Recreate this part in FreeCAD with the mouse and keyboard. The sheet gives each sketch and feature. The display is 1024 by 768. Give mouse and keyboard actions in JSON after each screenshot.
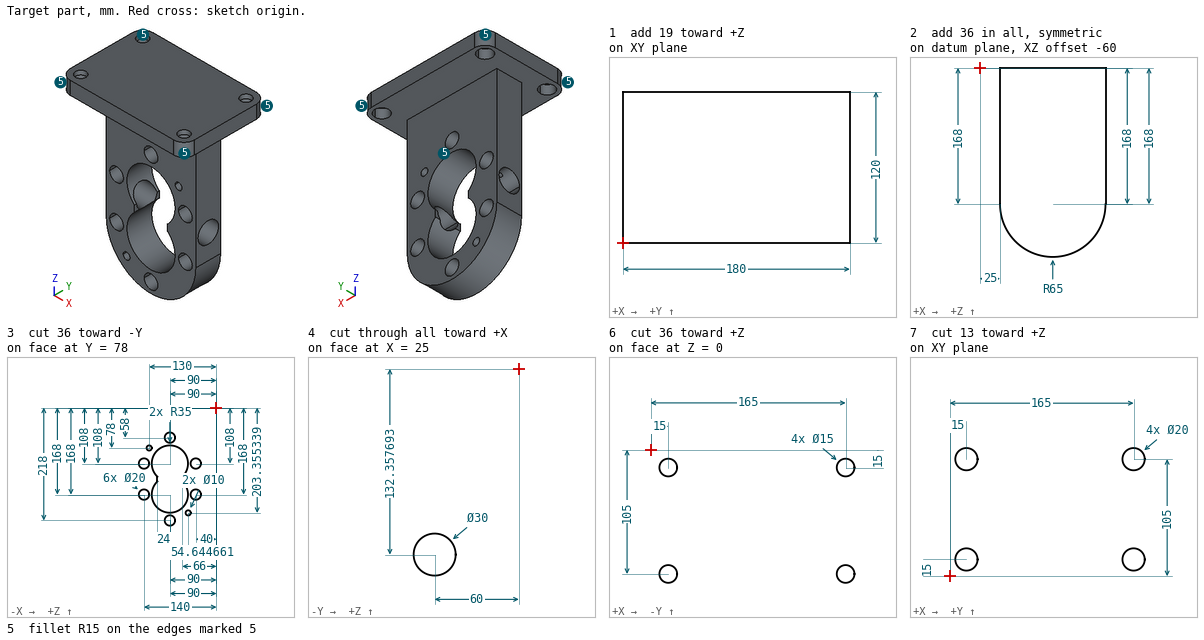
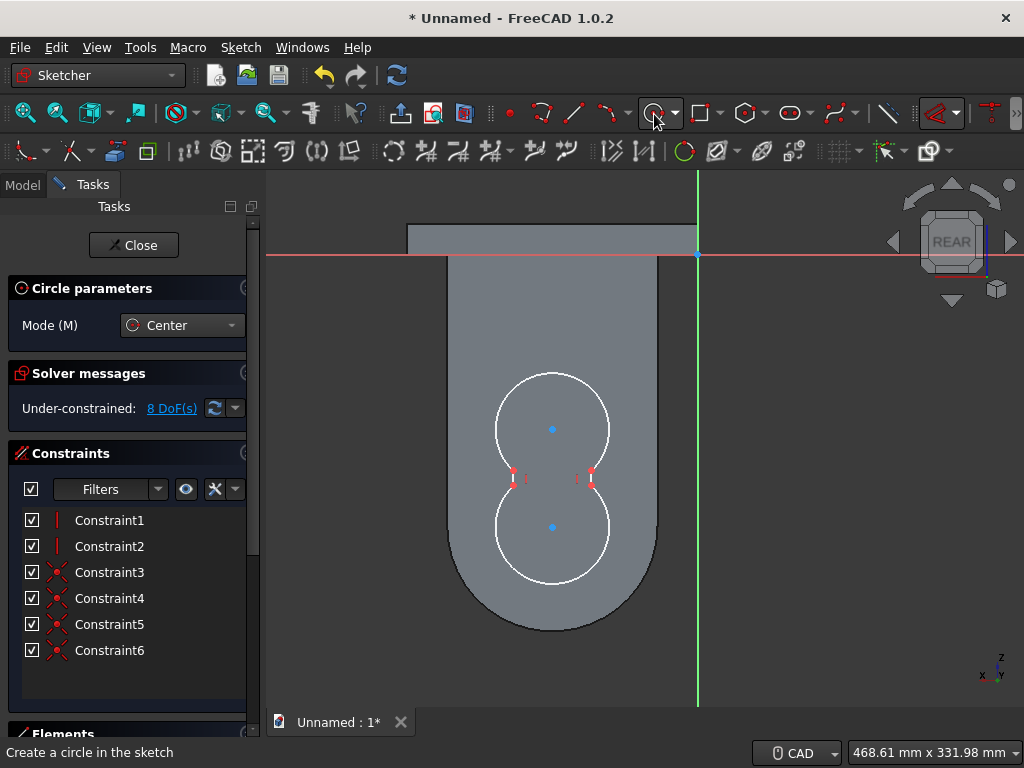
{"action": "scroll", "coordinate": [552, 607], "scroll_direction": "up", "scroll_amount": 2}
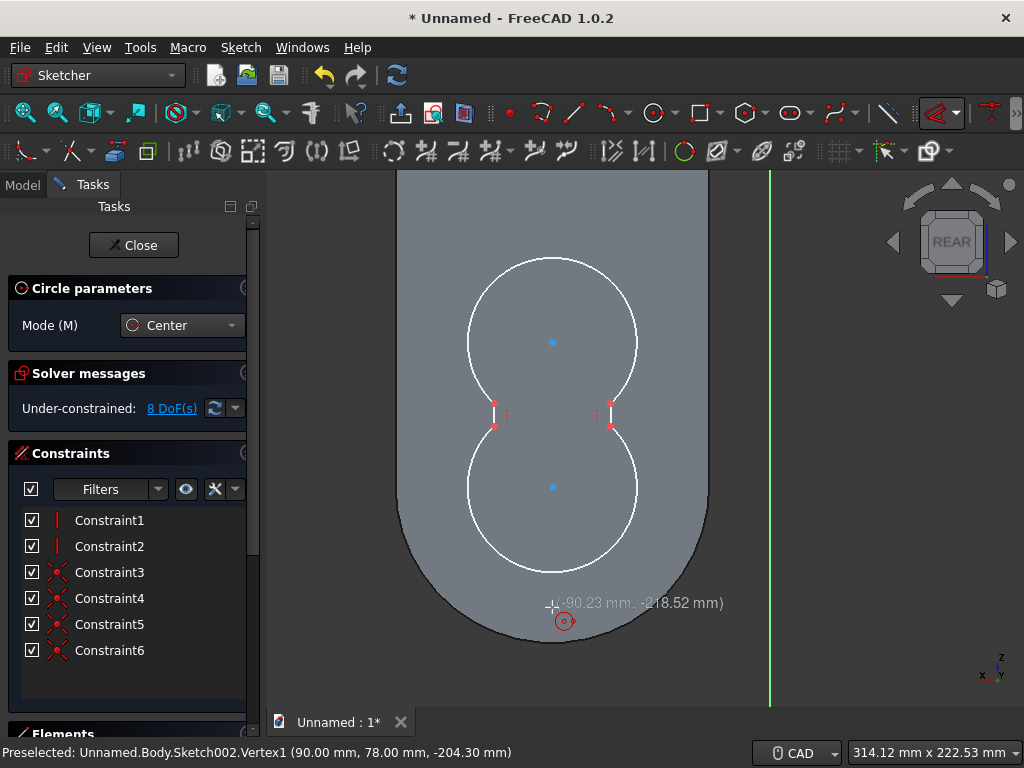
{"action": "left_click", "coordinate": [552, 607]}
{"action": "left_click", "coordinate": [569, 590]}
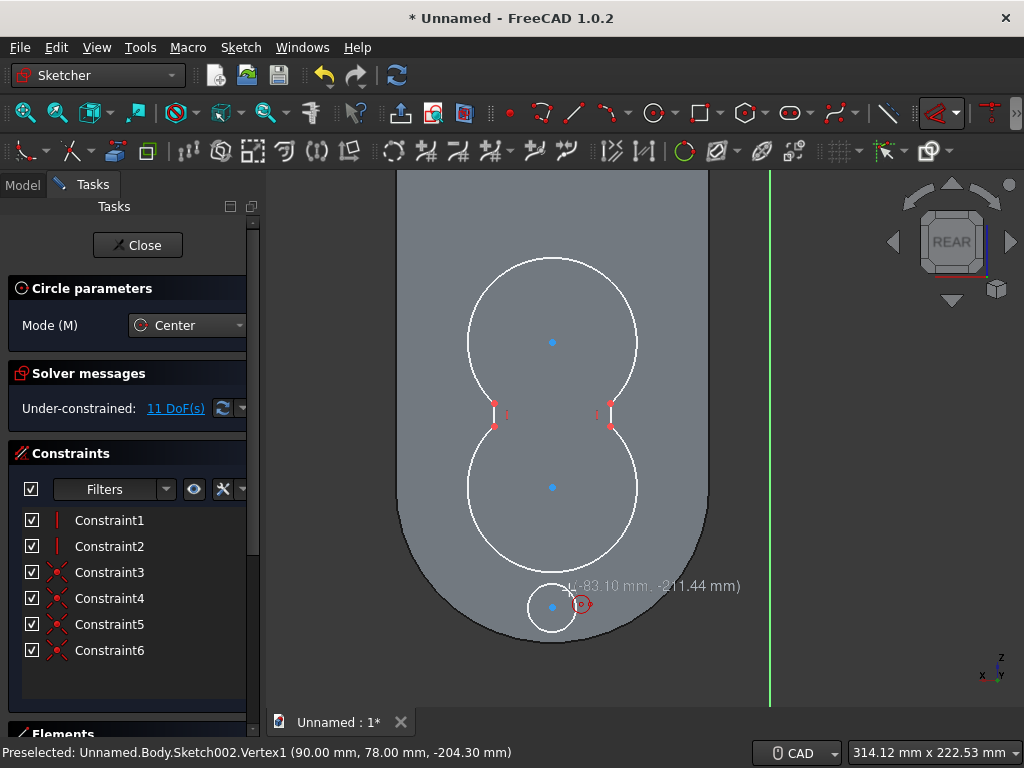
{"action": "left_click", "coordinate": [432, 486]}
{"action": "left_click", "coordinate": [449, 469]}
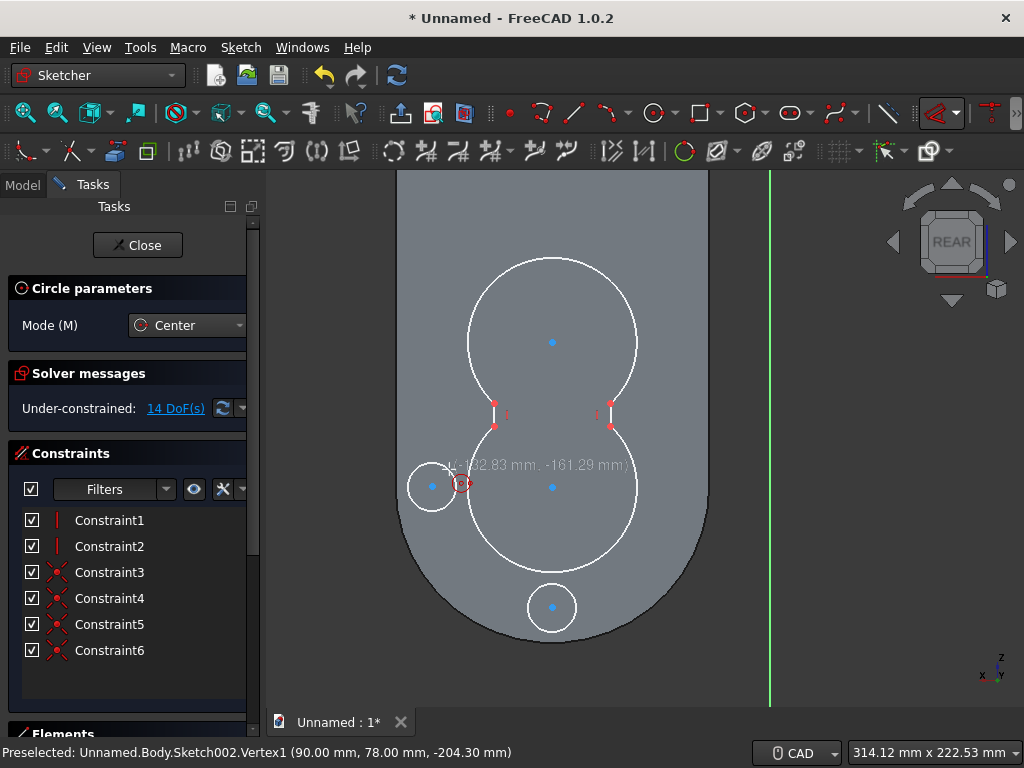
{"action": "left_click", "coordinate": [673, 486]}
{"action": "left_click", "coordinate": [690, 469]}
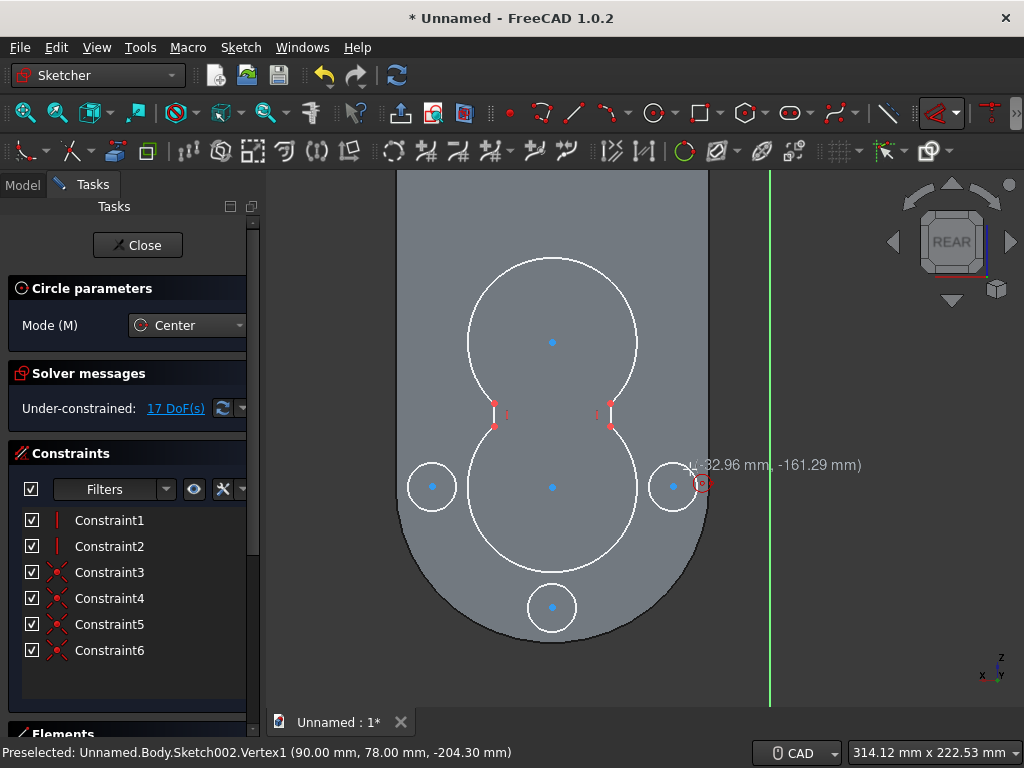
{"action": "left_click", "coordinate": [552, 221]}
{"action": "left_click", "coordinate": [569, 204]}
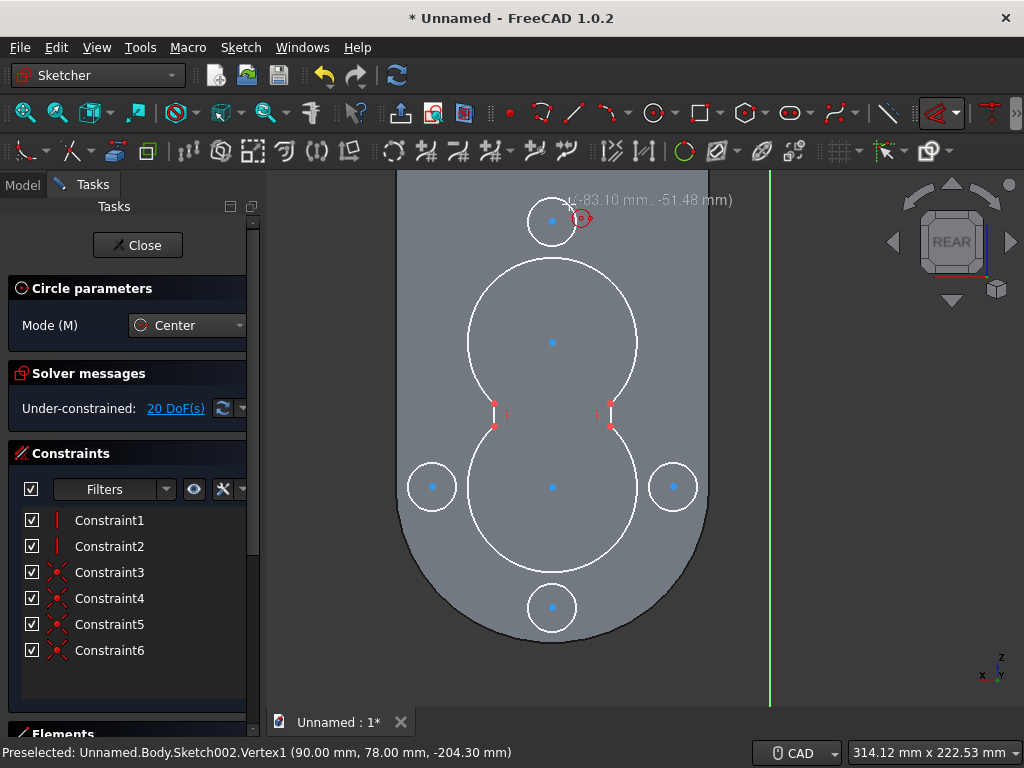
{"action": "left_click", "coordinate": [673, 341]}
{"action": "left_click", "coordinate": [690, 324]}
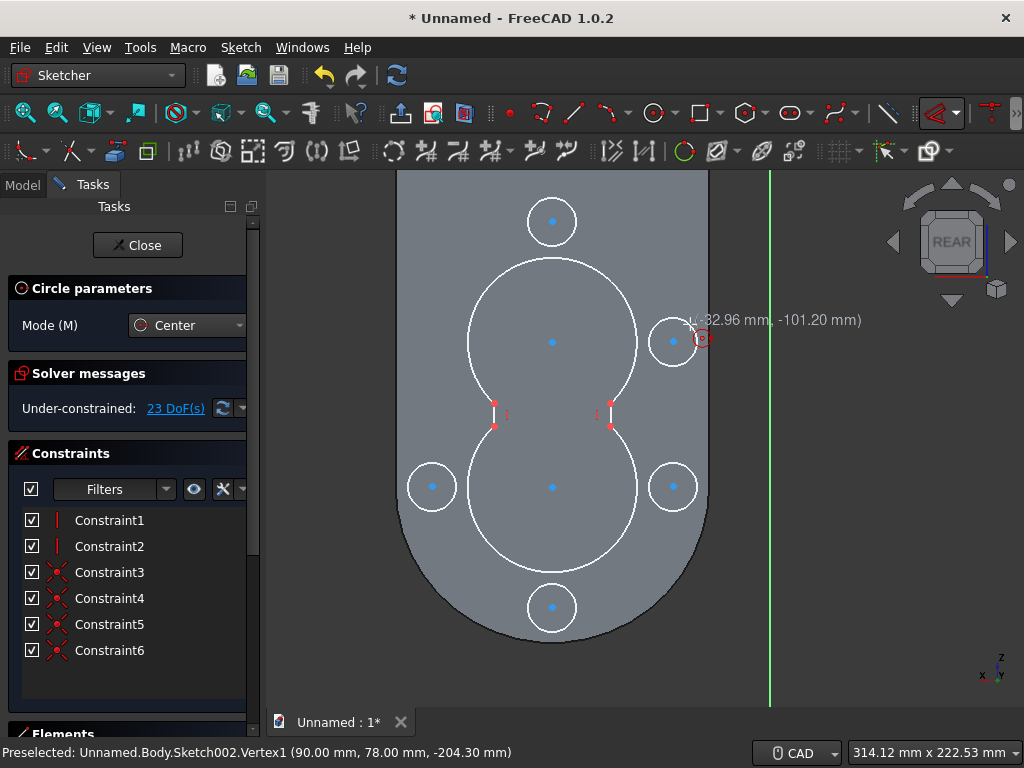
{"action": "left_click", "coordinate": [432, 341]}
{"action": "left_click", "coordinate": [449, 324]}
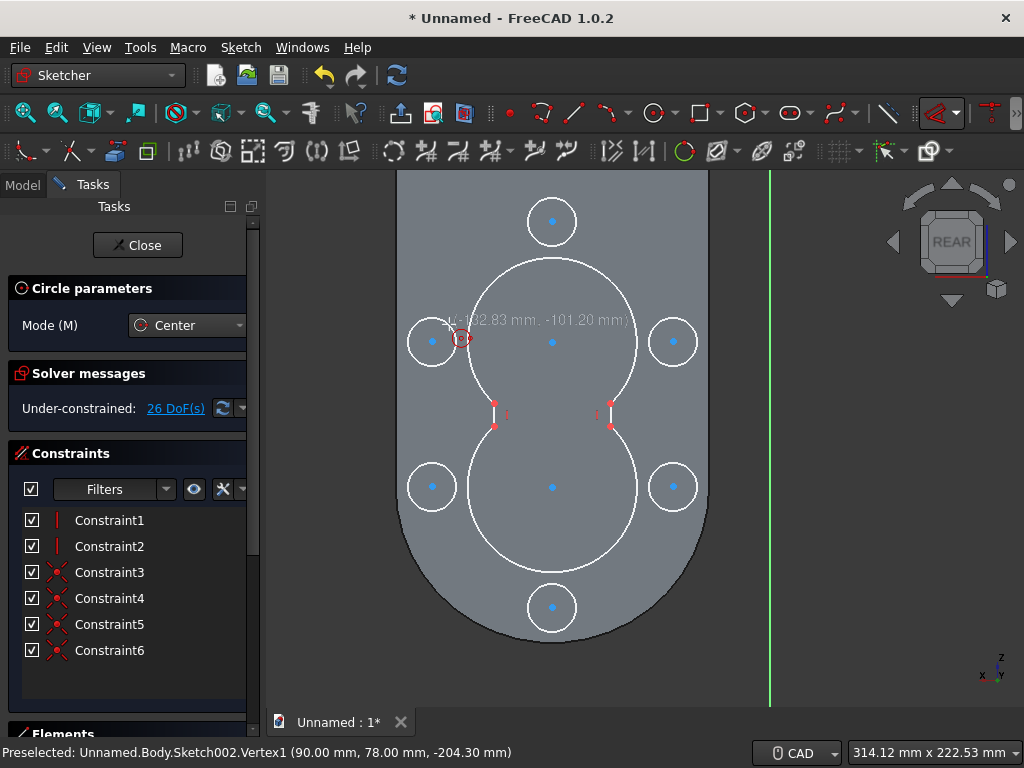
{"action": "scroll", "coordinate": [638, 572], "scroll_direction": "up", "scroll_amount": 4}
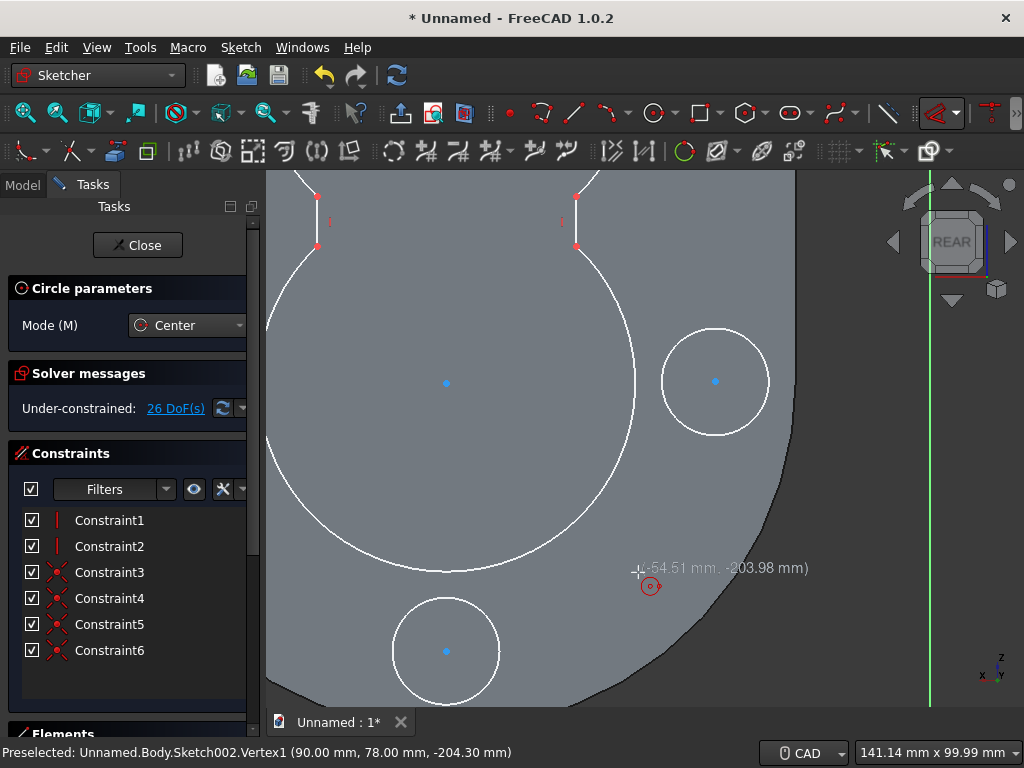
{"action": "left_click", "coordinate": [637, 570]}
{"action": "left_click", "coordinate": [656, 551]}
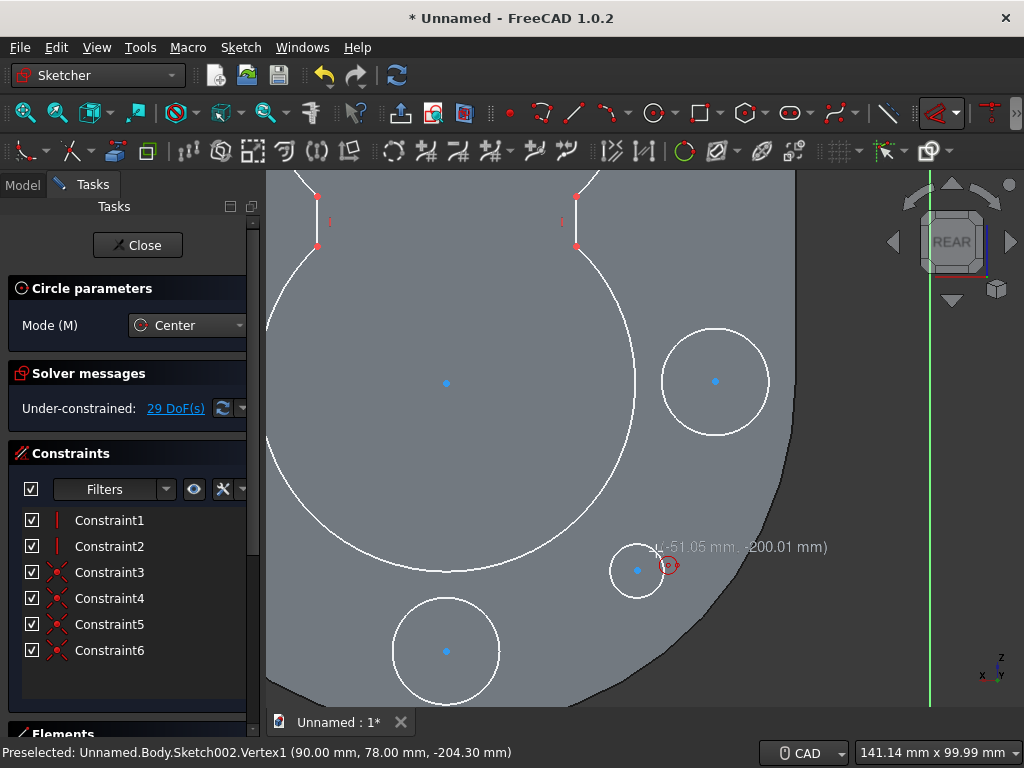
{"action": "scroll", "coordinate": [598, 589], "scroll_direction": "down", "scroll_amount": 6}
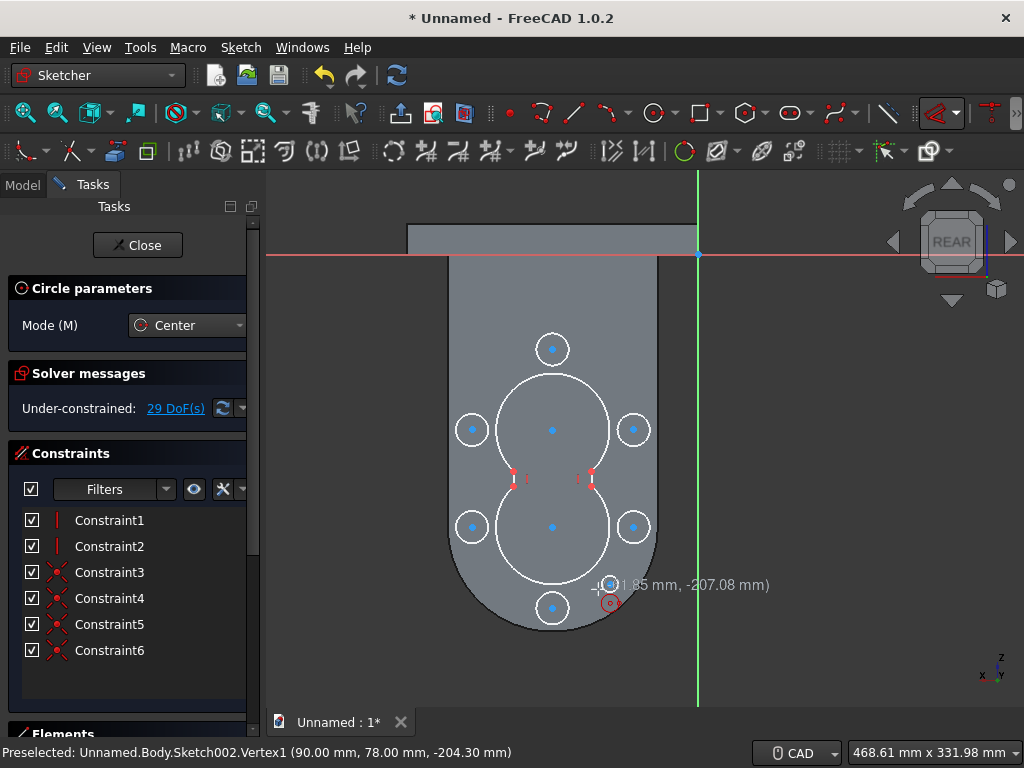
{"action": "scroll", "coordinate": [488, 381], "scroll_direction": "up", "scroll_amount": 6}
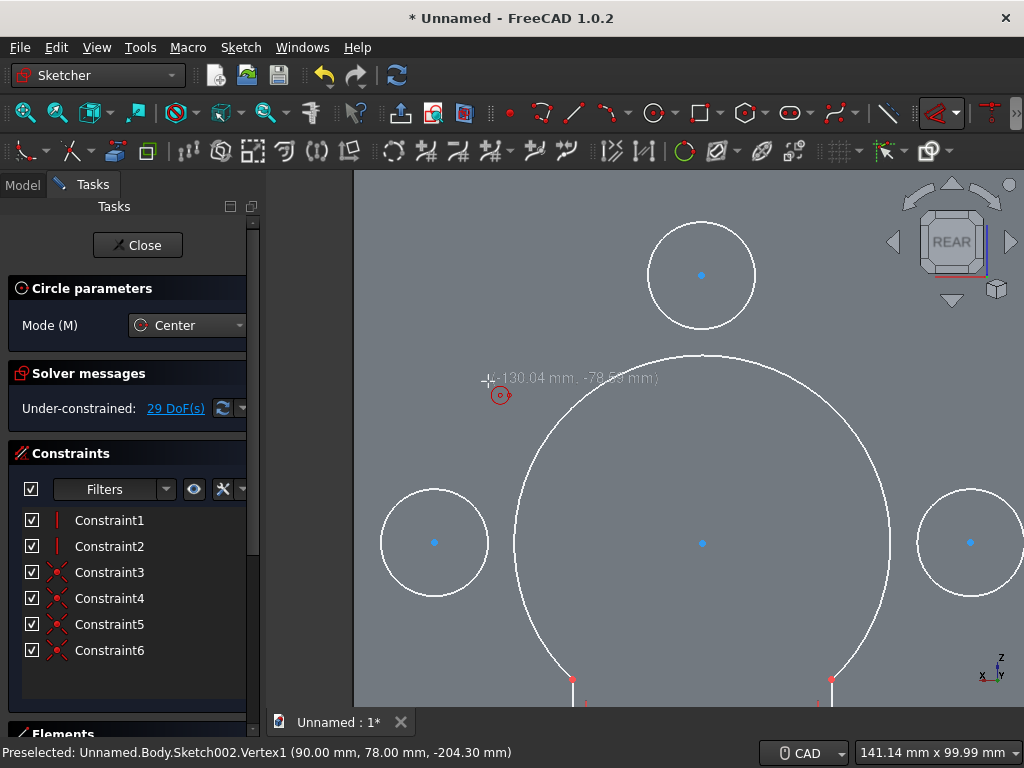
{"action": "left_click", "coordinate": [488, 380]}
{"action": "left_click", "coordinate": [507, 361]}
{"action": "key", "text": "Escape"}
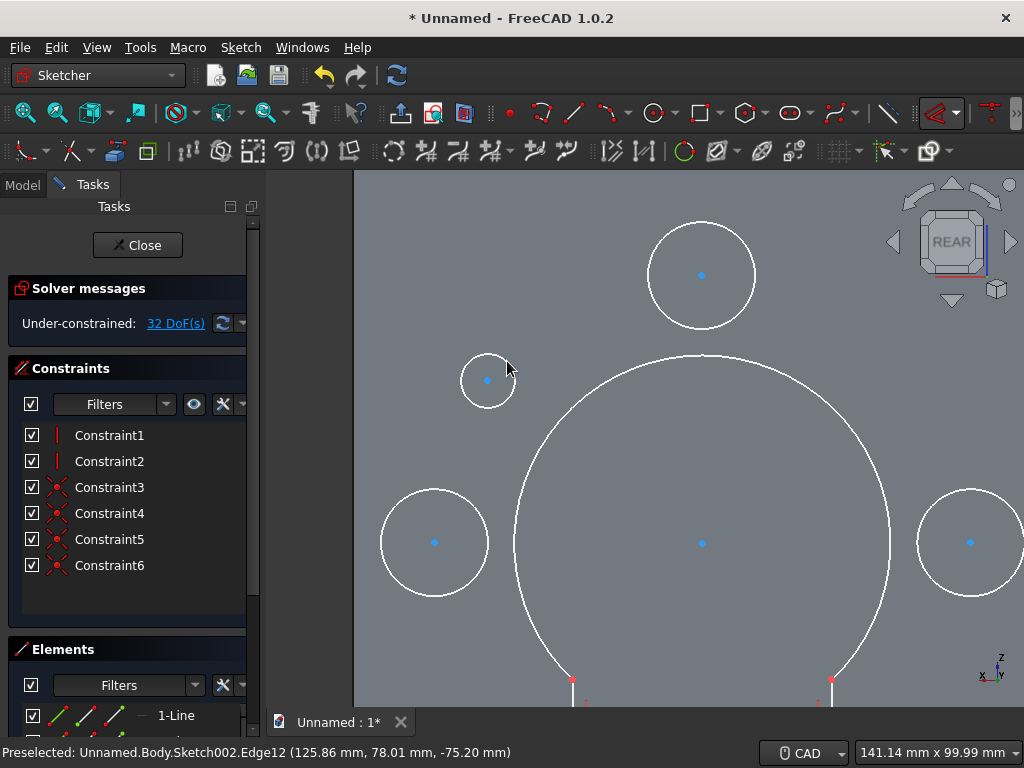
{"action": "left_click", "coordinate": [856, 435]}